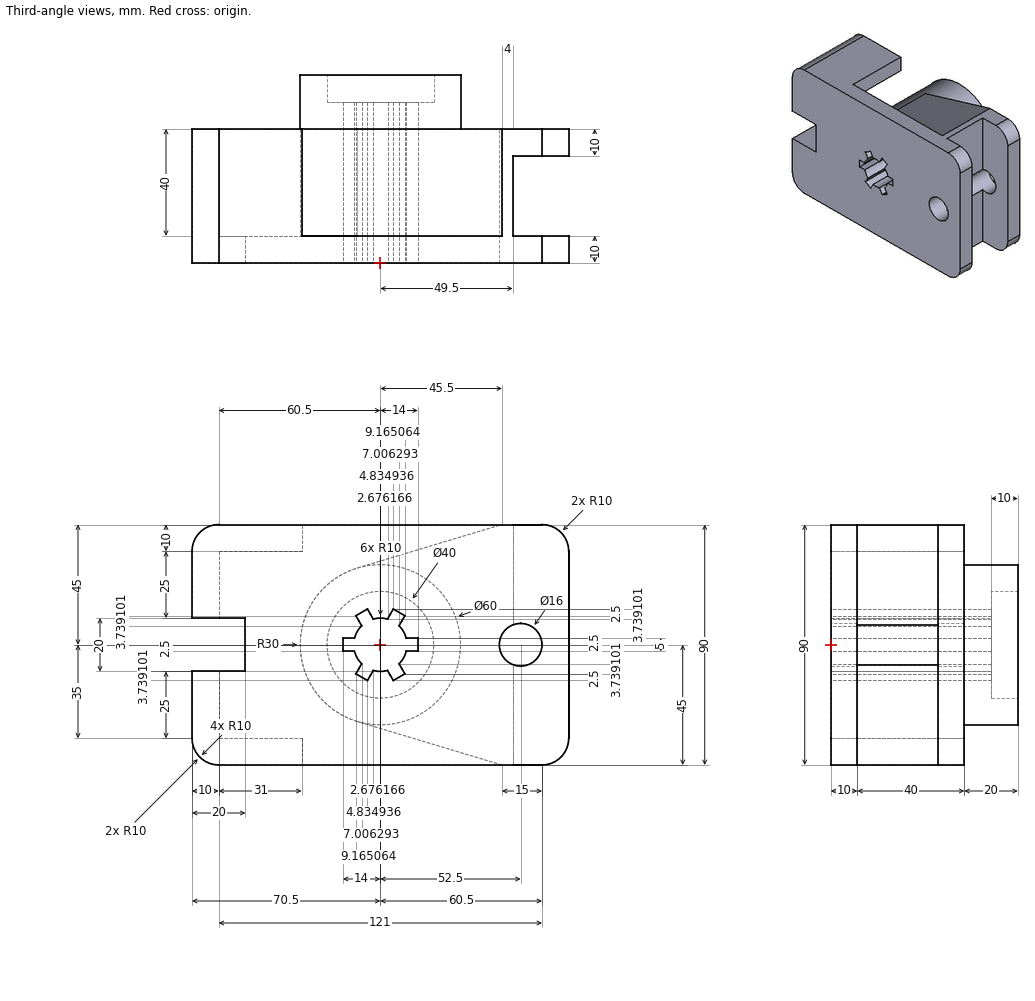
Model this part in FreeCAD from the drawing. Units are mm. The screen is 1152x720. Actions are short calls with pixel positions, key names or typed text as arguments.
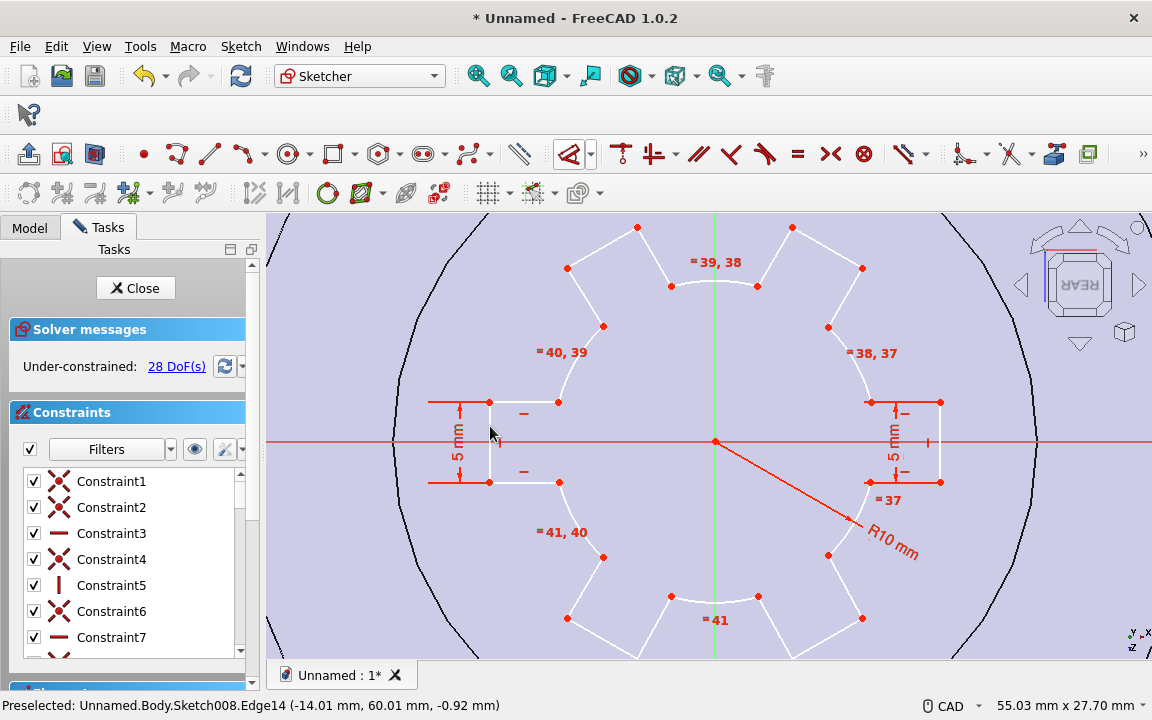
click(940, 483)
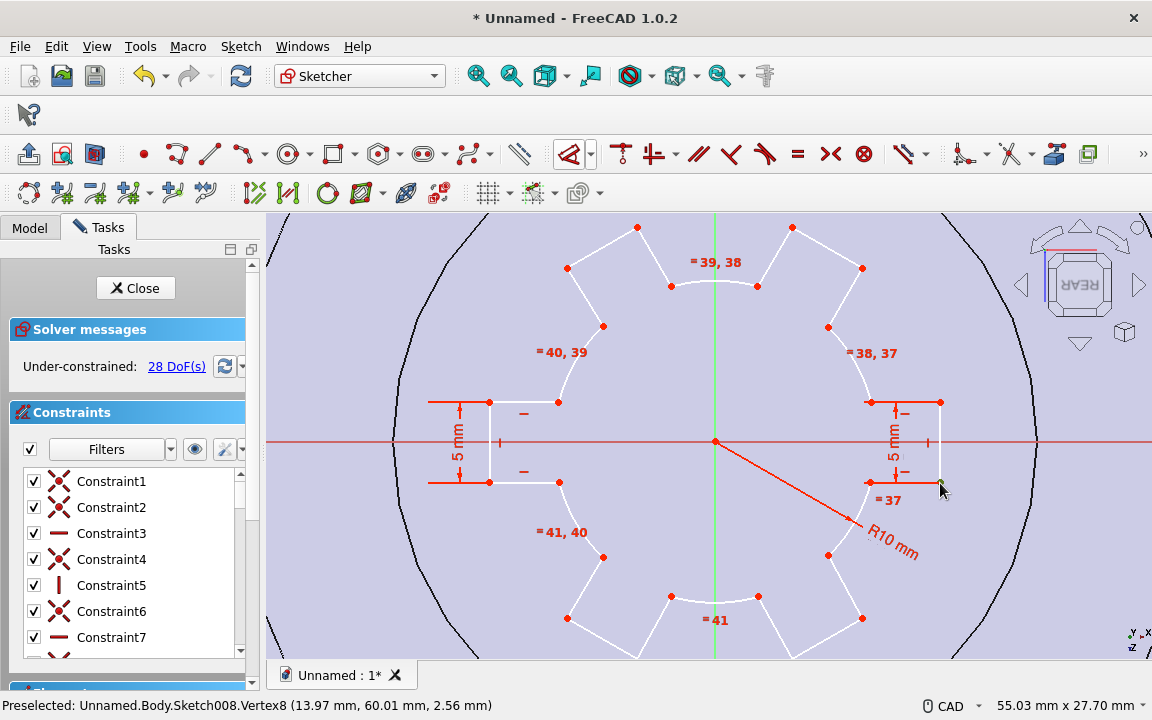
click(590, 154)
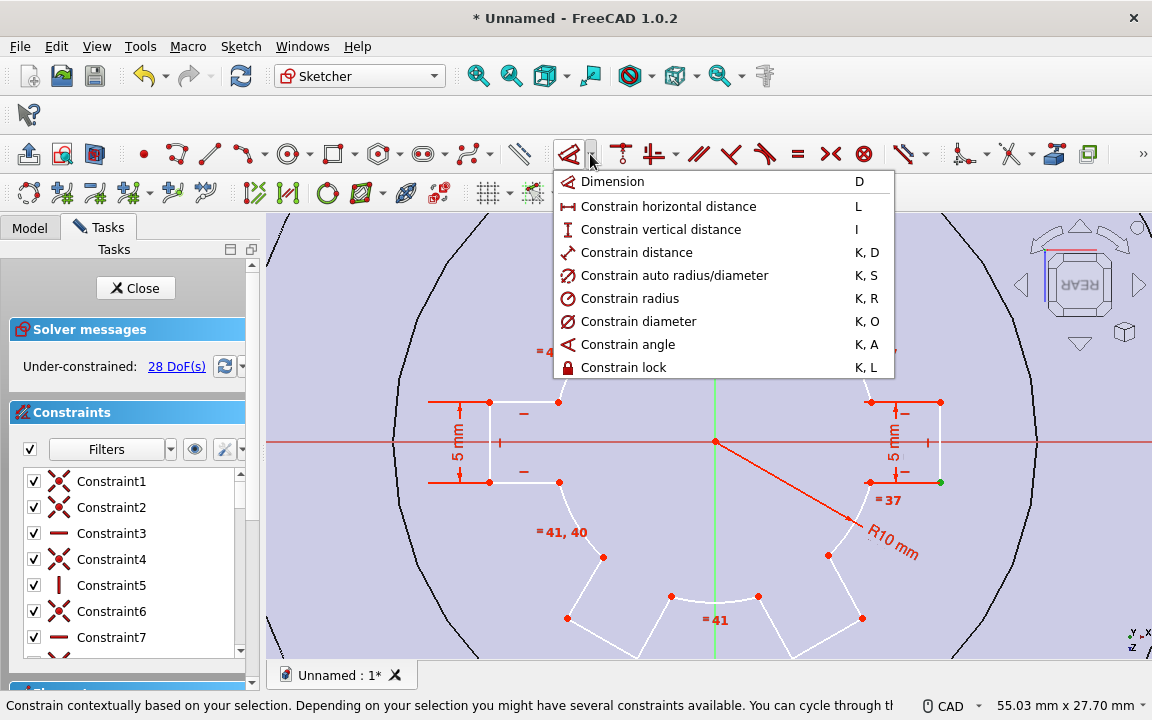
click(724, 206)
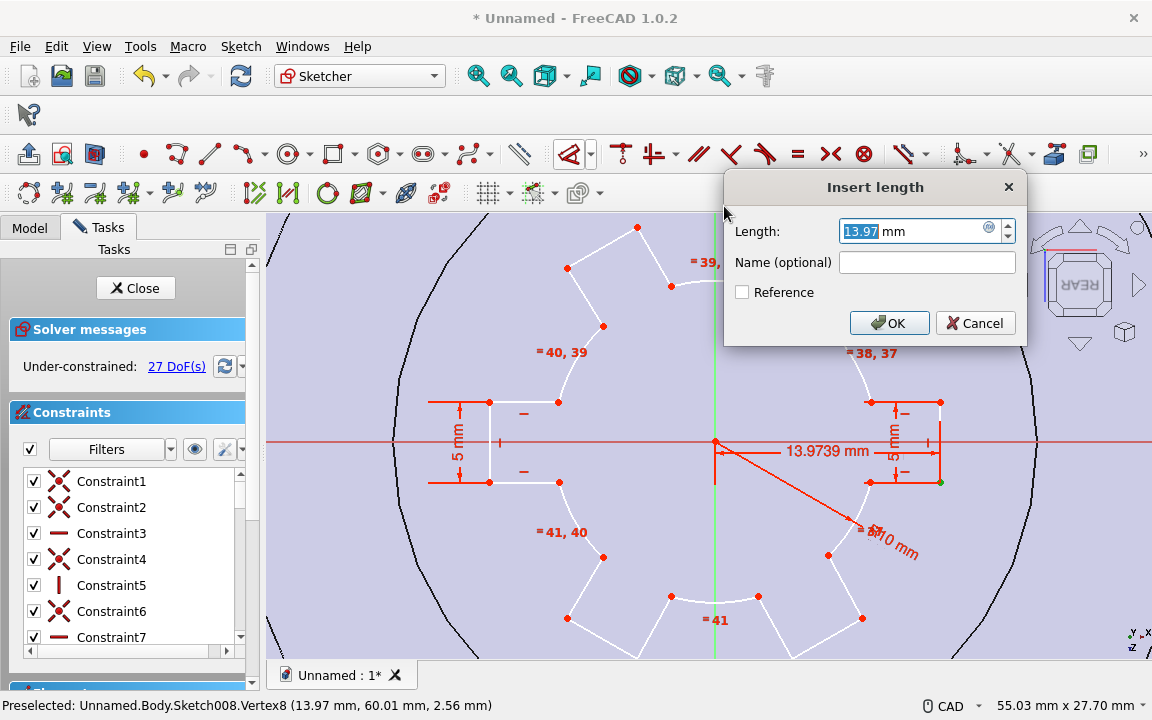
text(14)
key(Return)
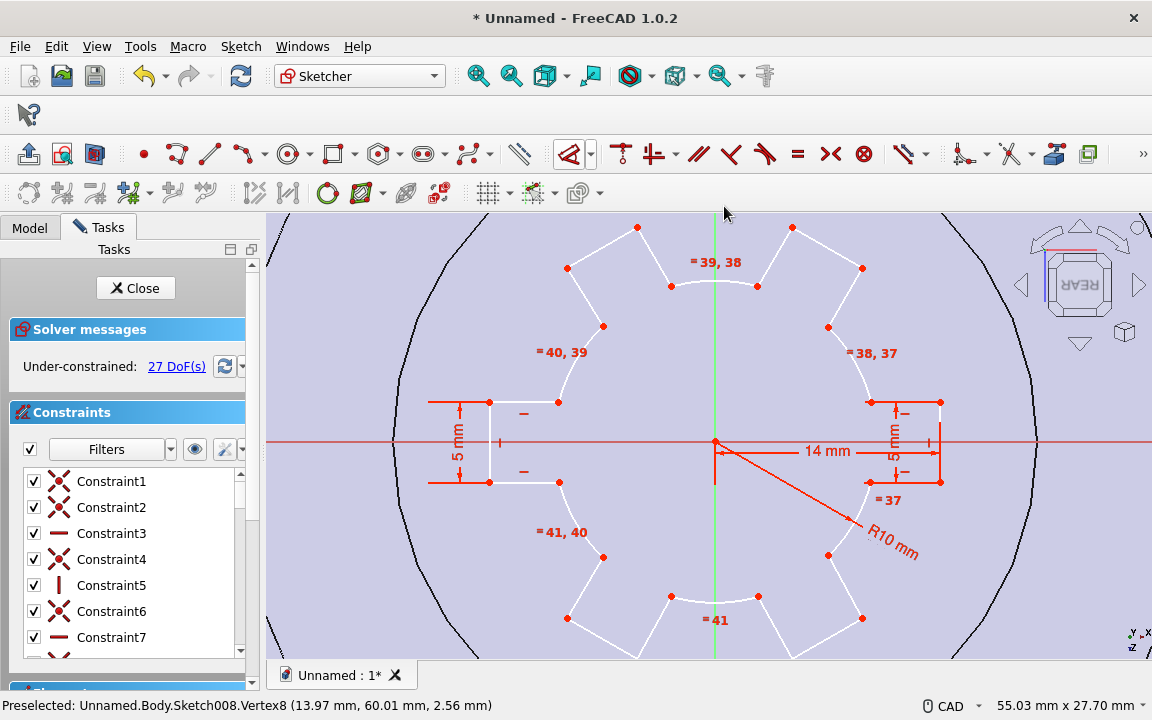
click(490, 402)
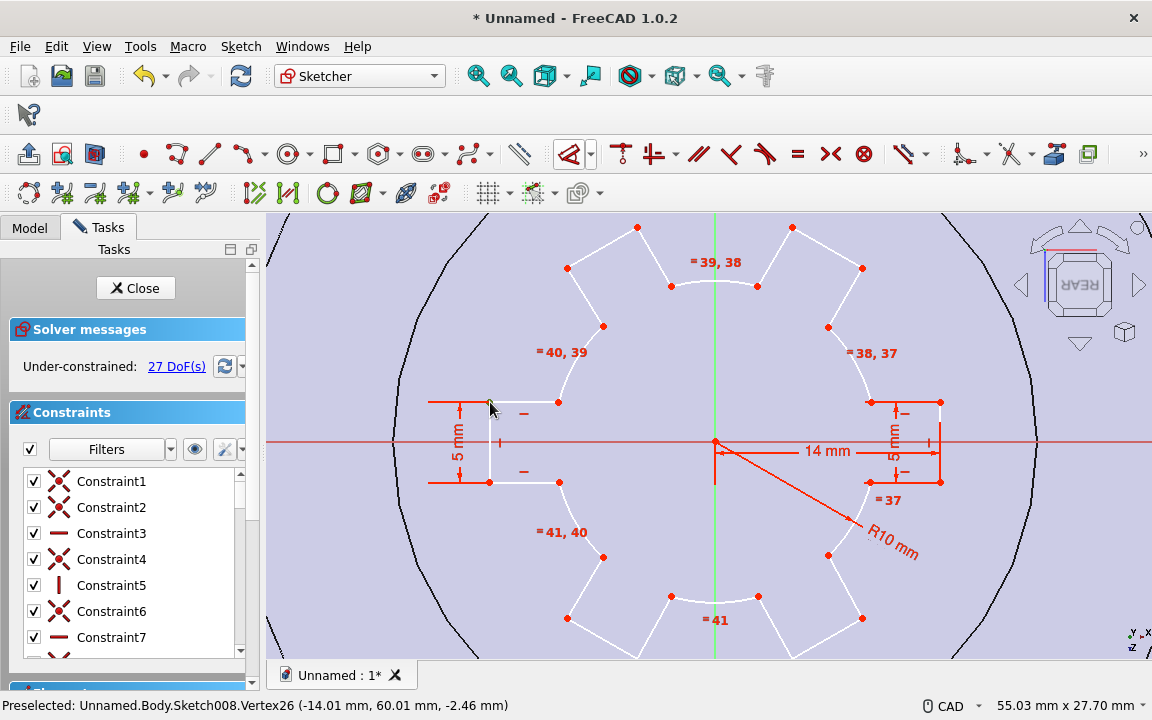
key(l)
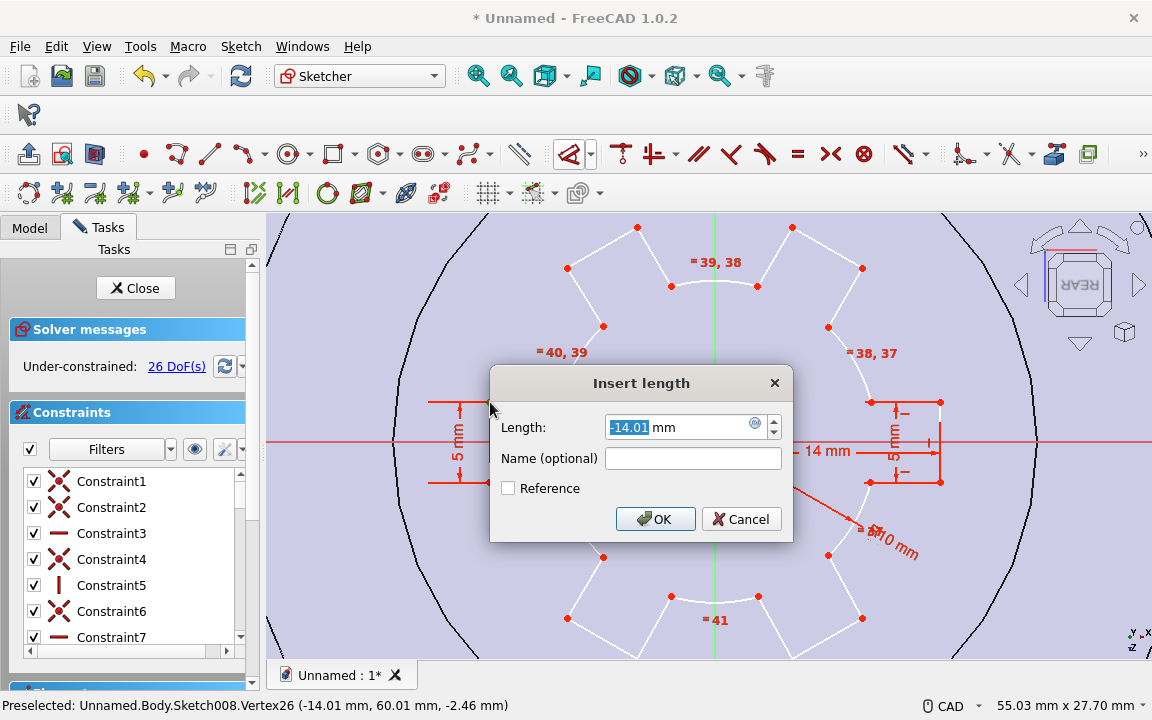
text(-14)
key(Return)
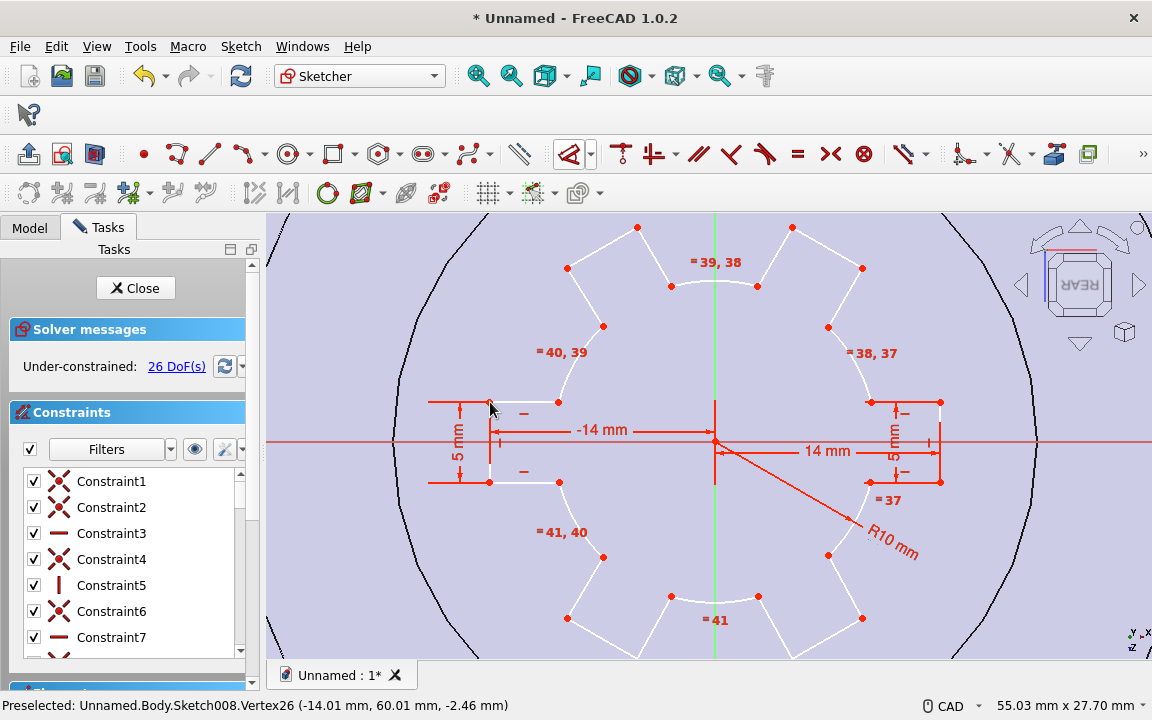
click(871, 483)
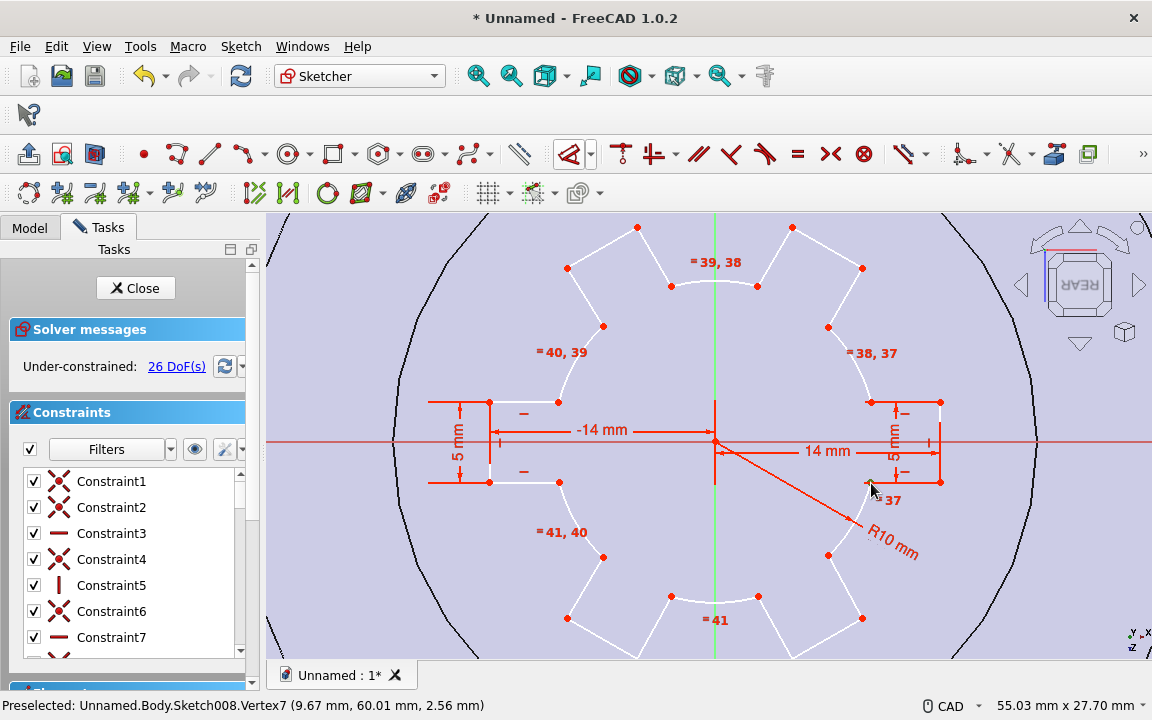
click(590, 154)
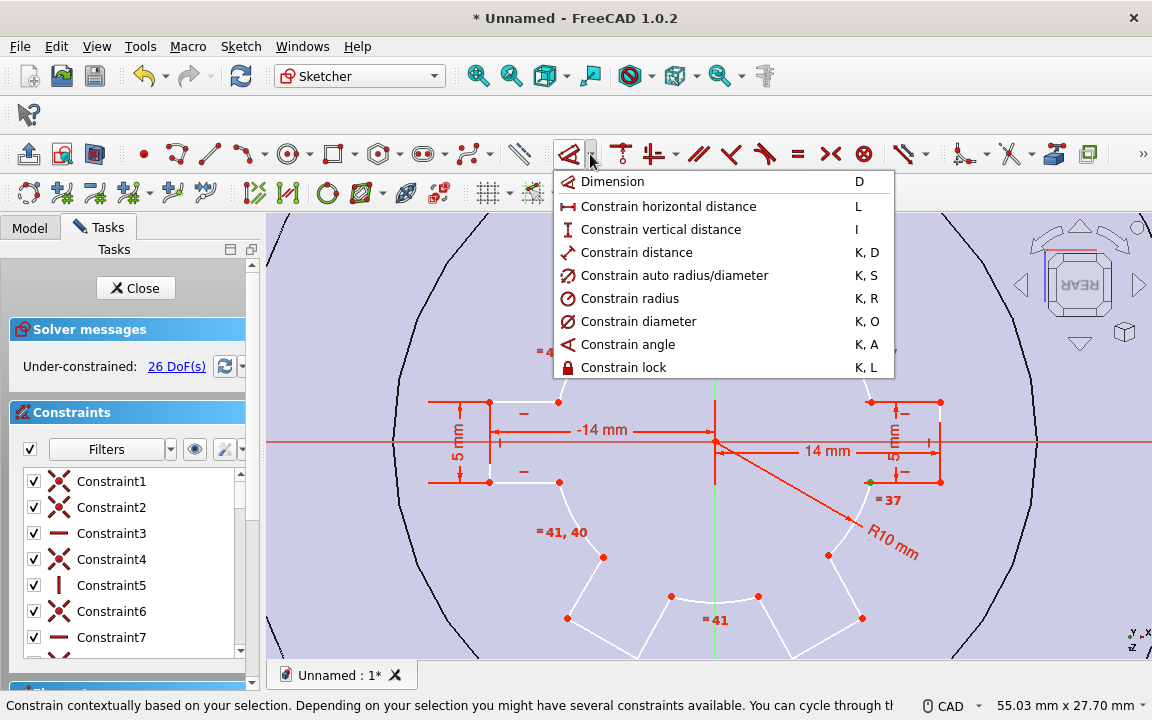
click(724, 230)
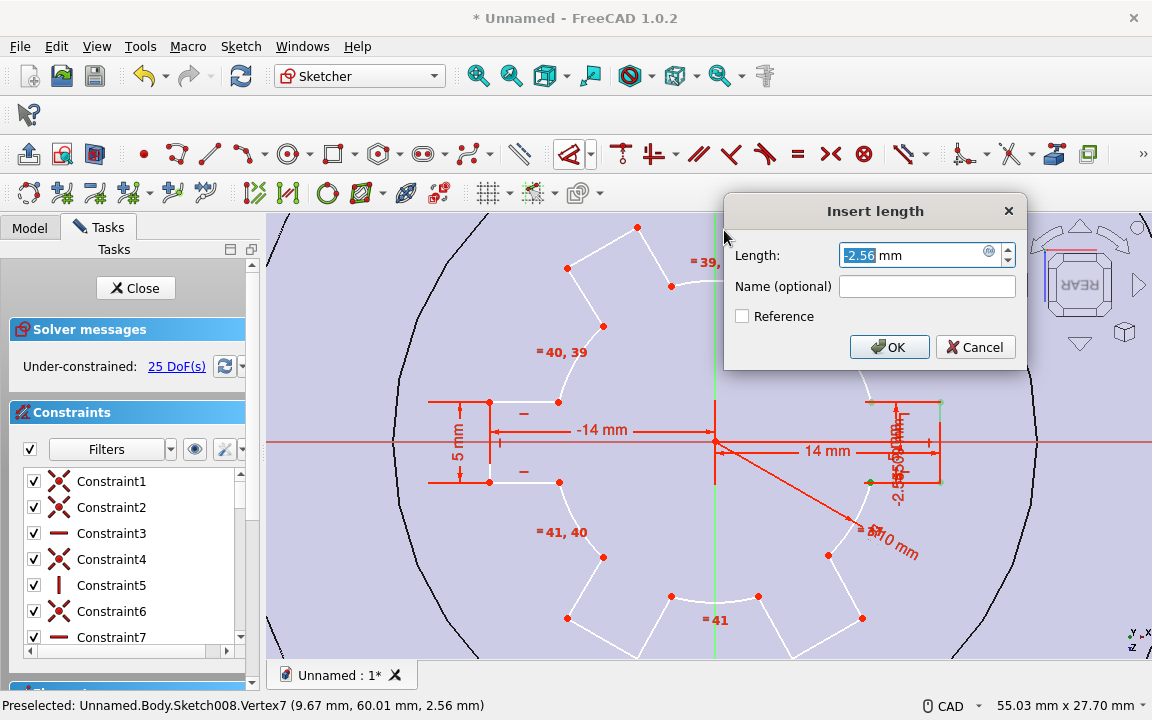
text(-2.5)
key(Return)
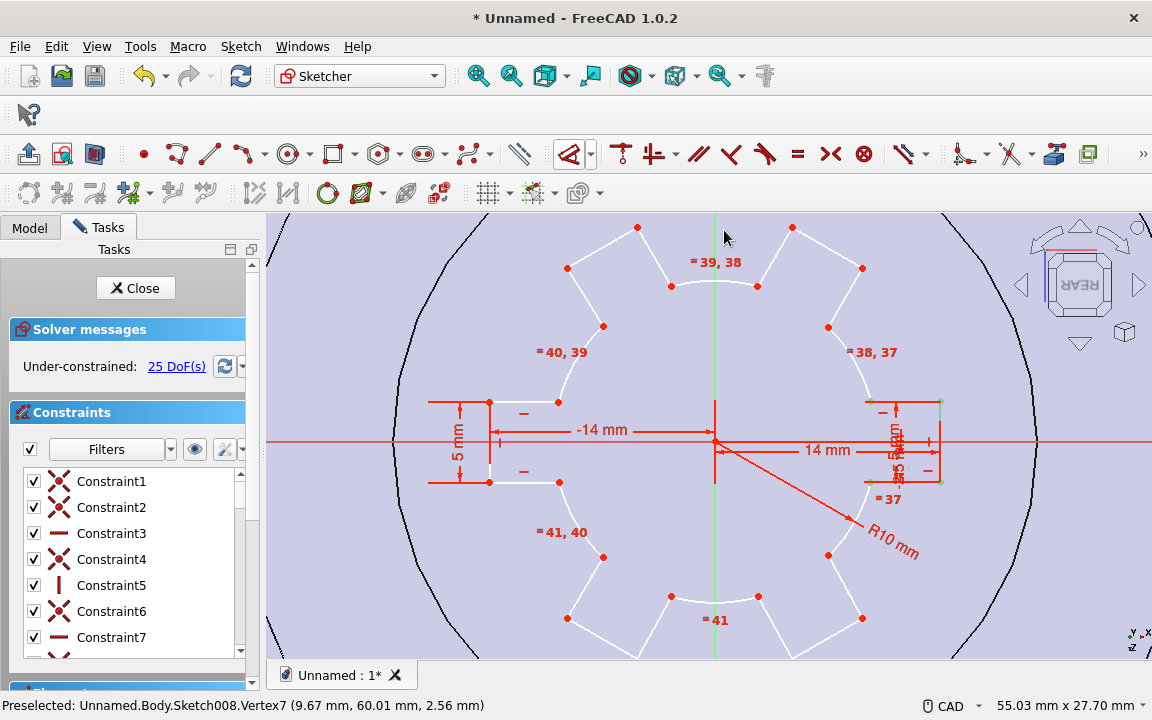
click(559, 402)